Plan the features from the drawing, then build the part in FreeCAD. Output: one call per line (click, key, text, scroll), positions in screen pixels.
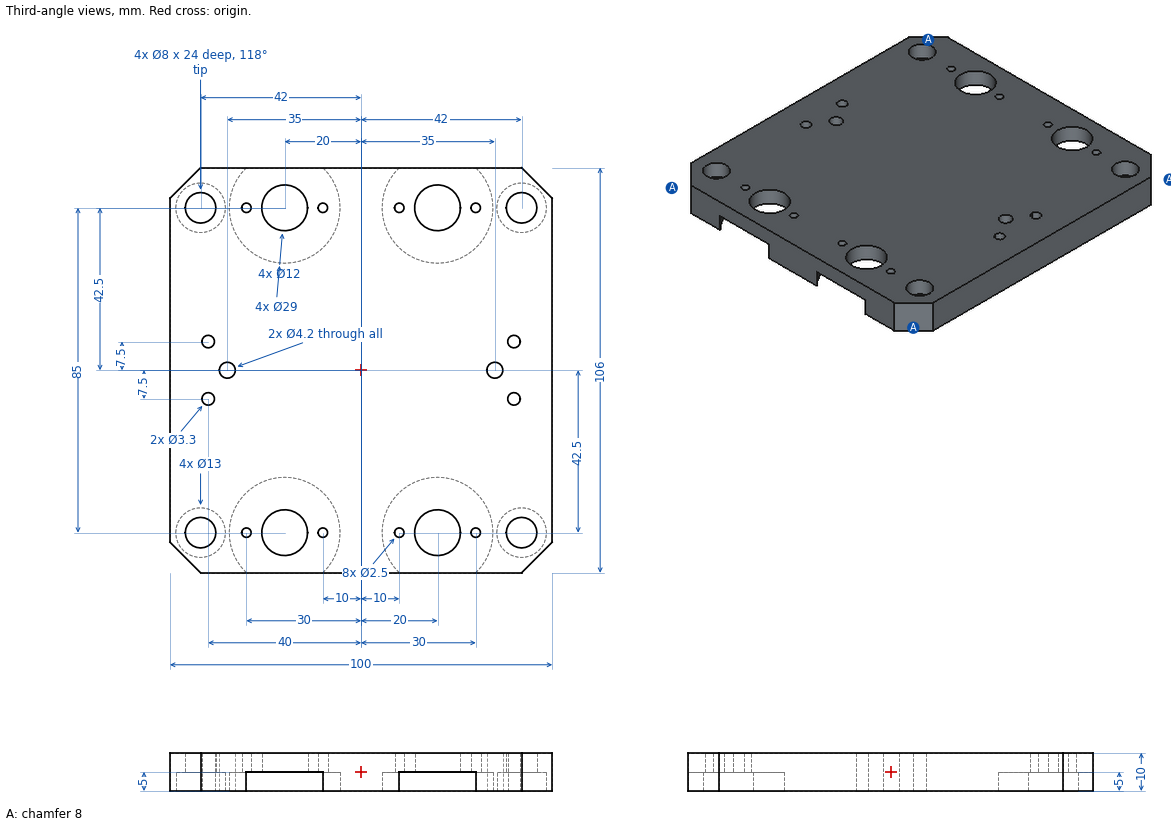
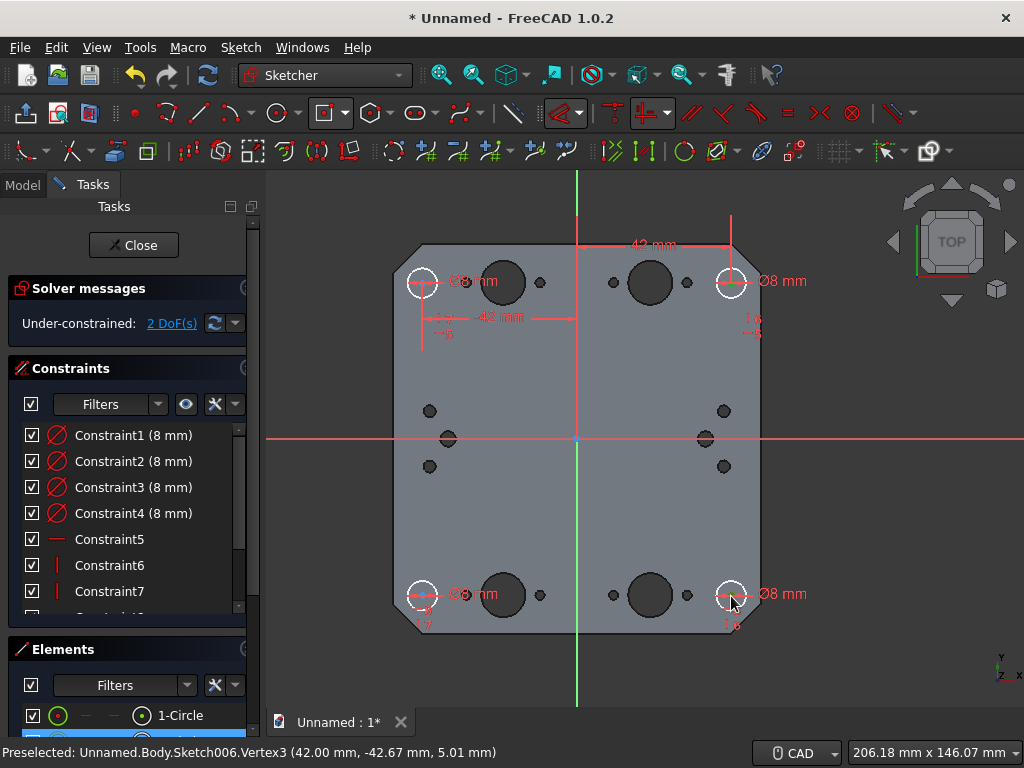
key(i)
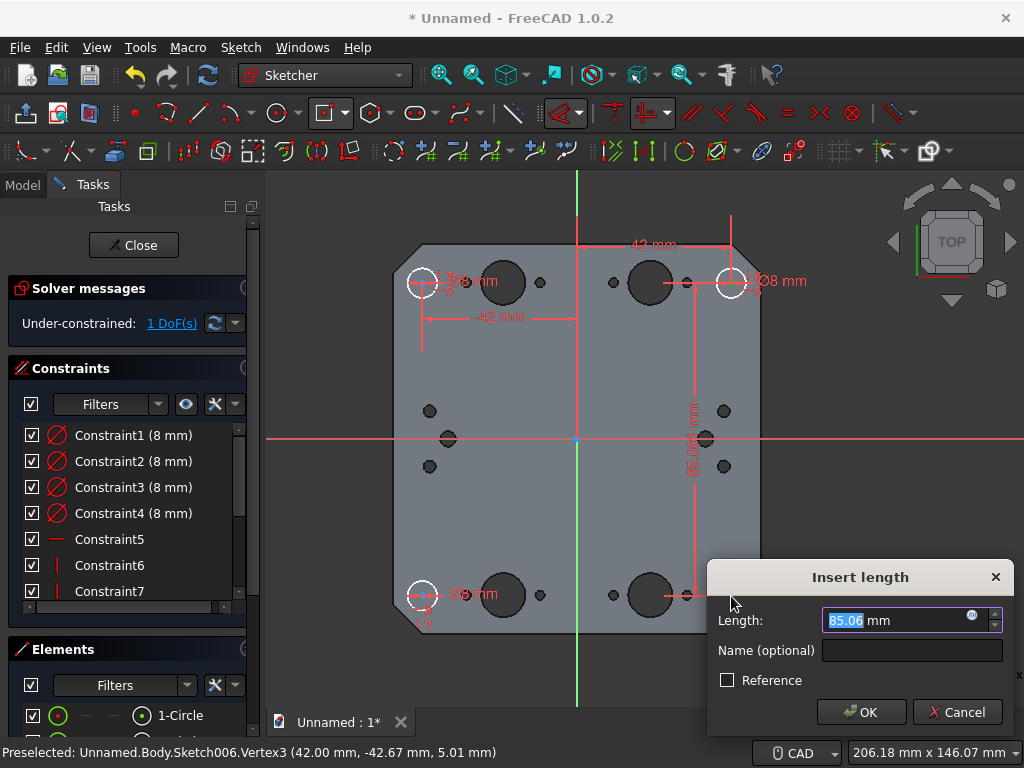
text(85)
key(Return)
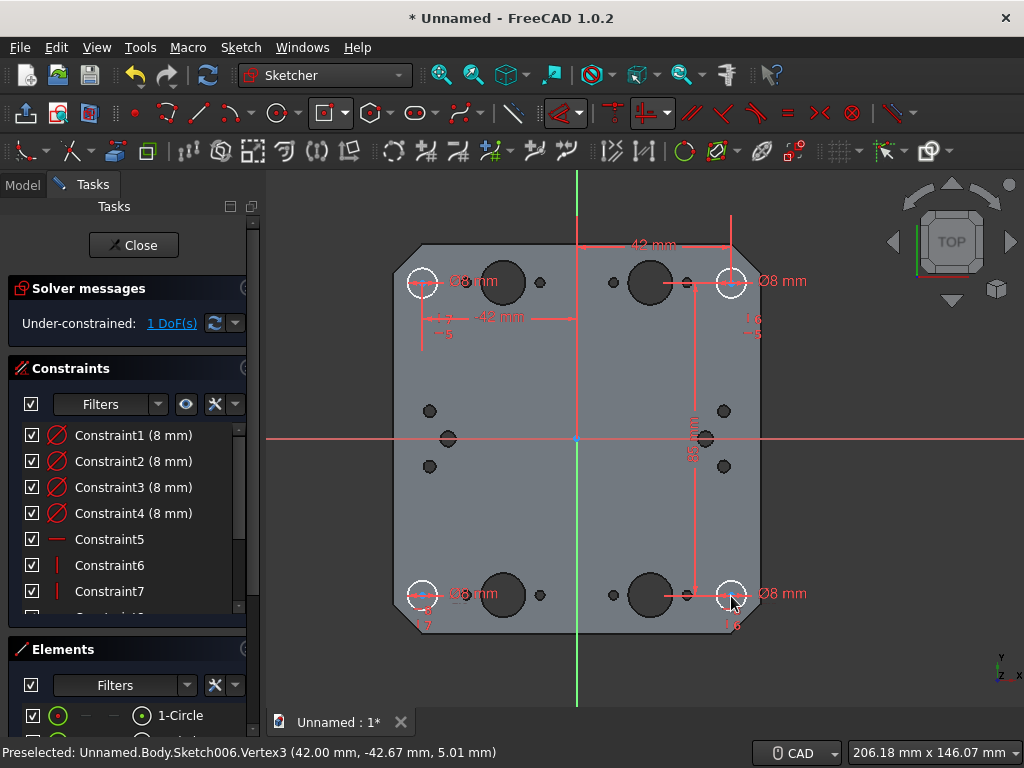
click(422, 283)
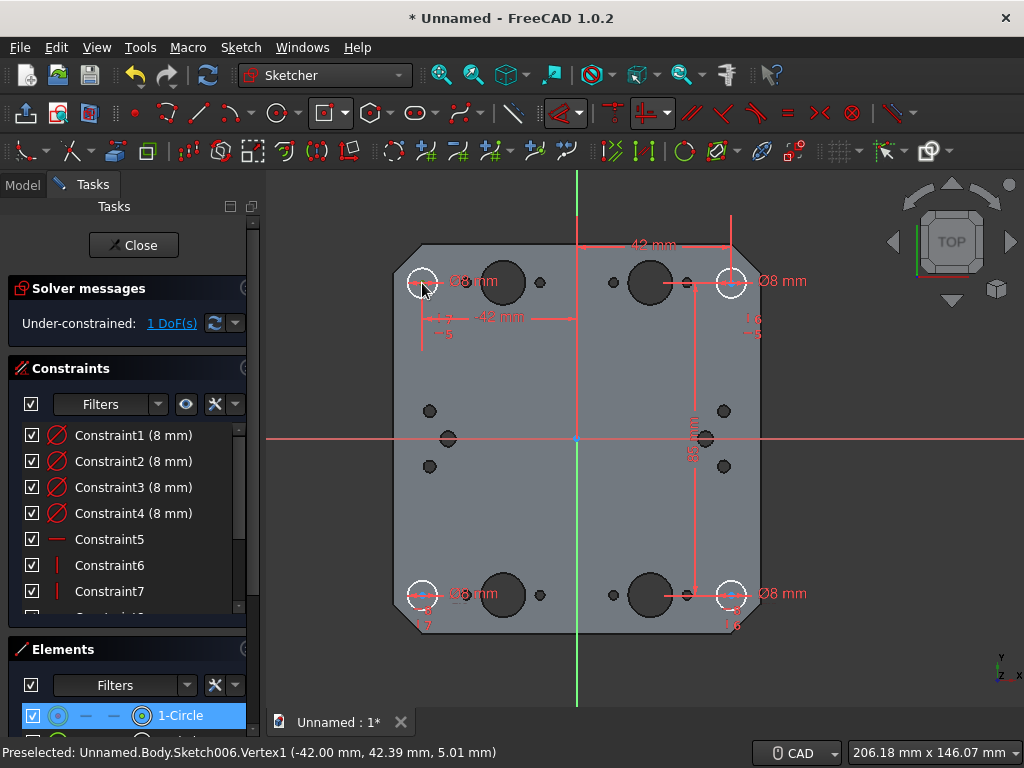
click(582, 114)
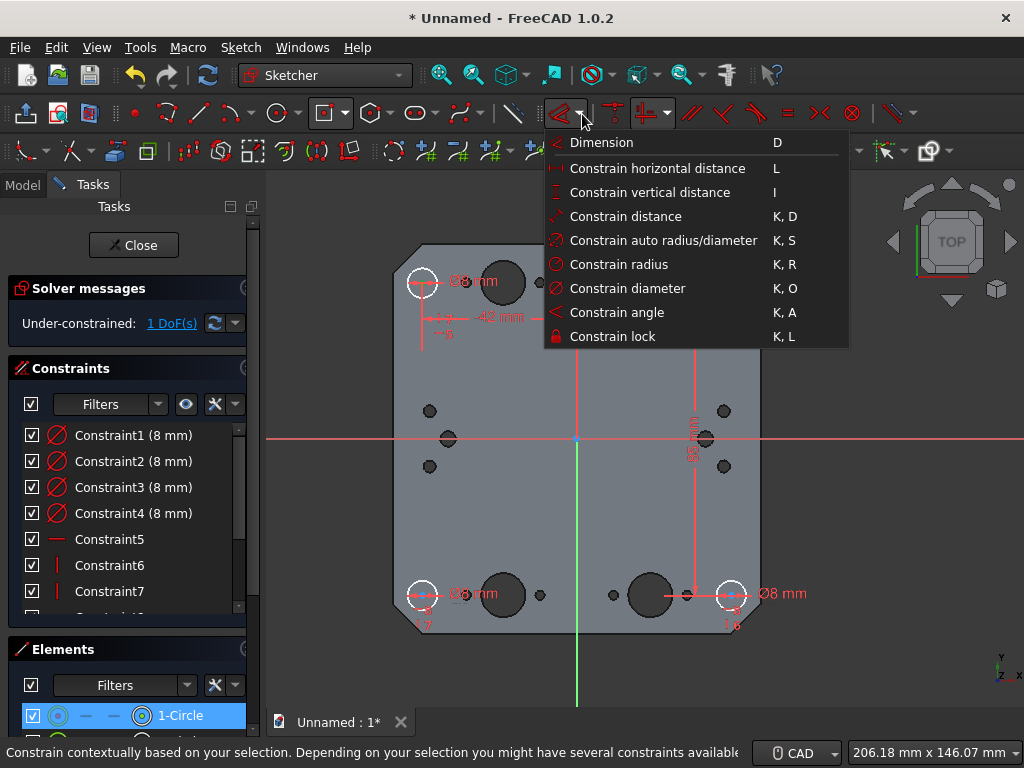
click(697, 192)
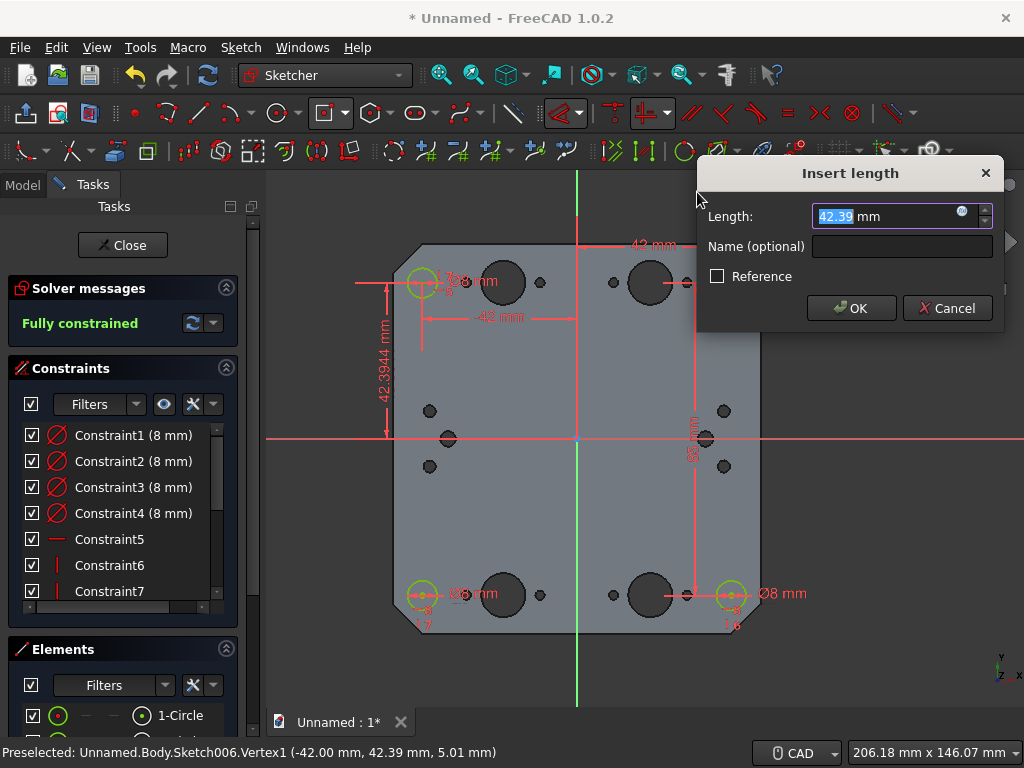
text(42.5)
key(Return)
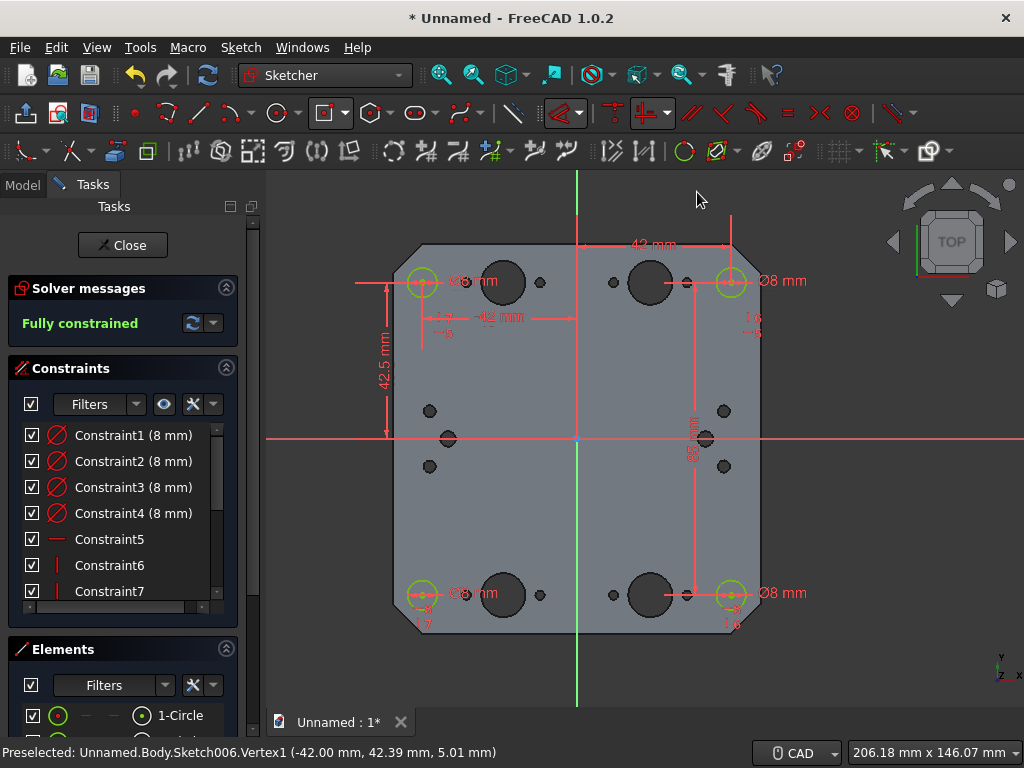
click(123, 245)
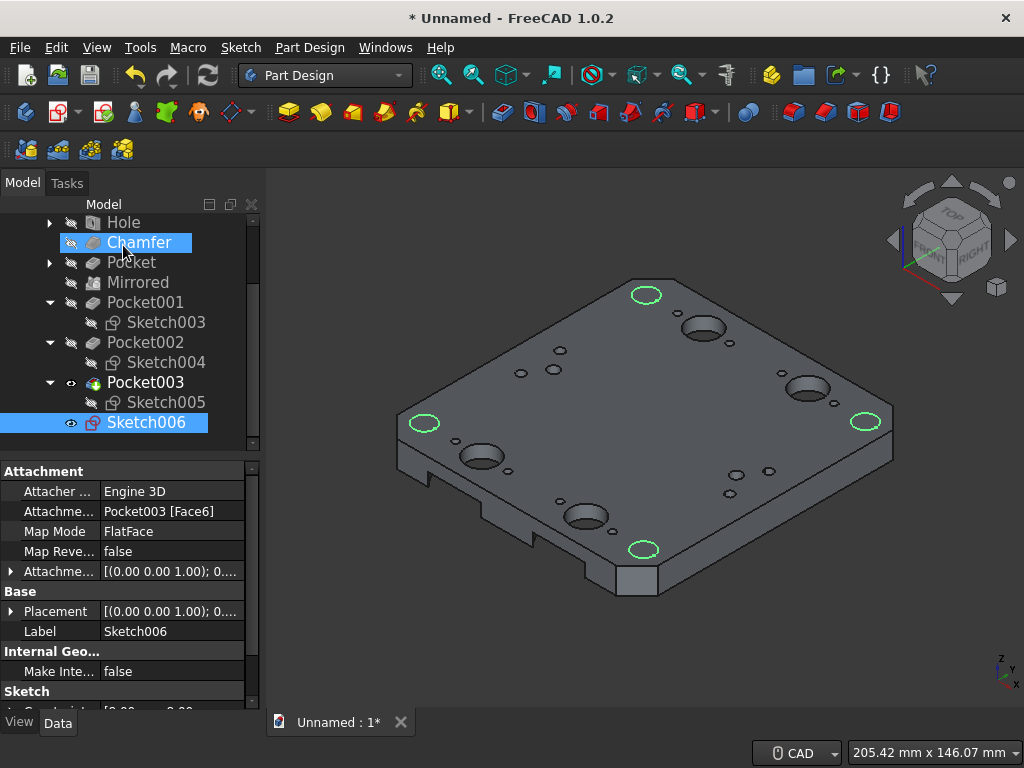
click(536, 112)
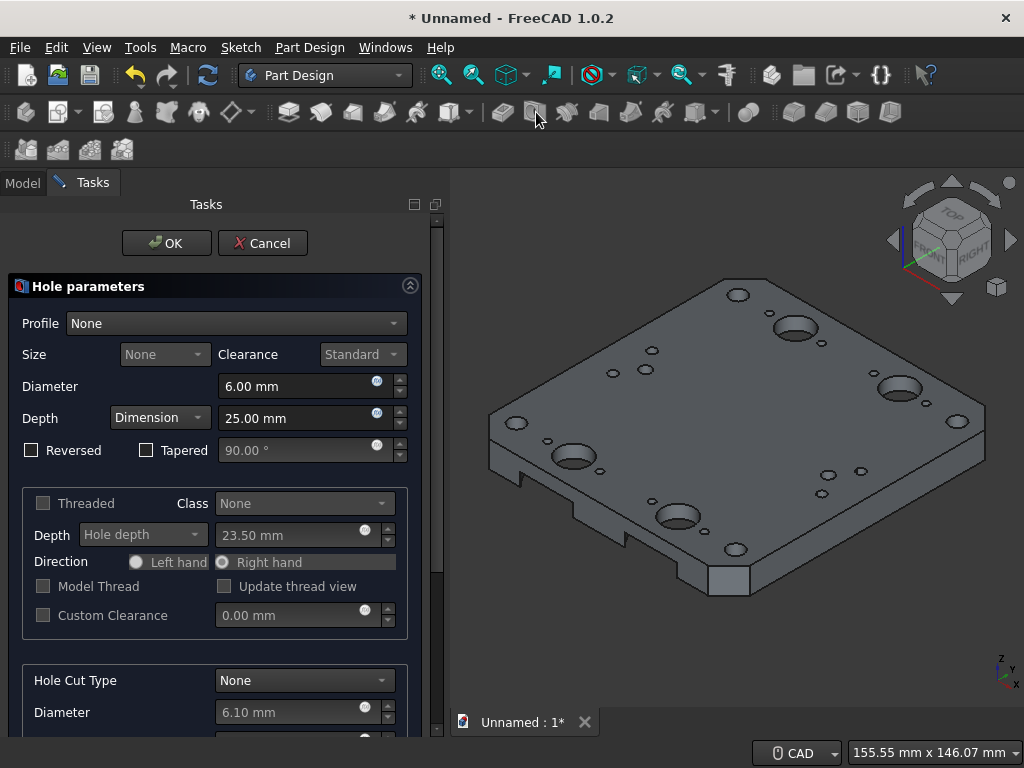
triple_click(305, 386)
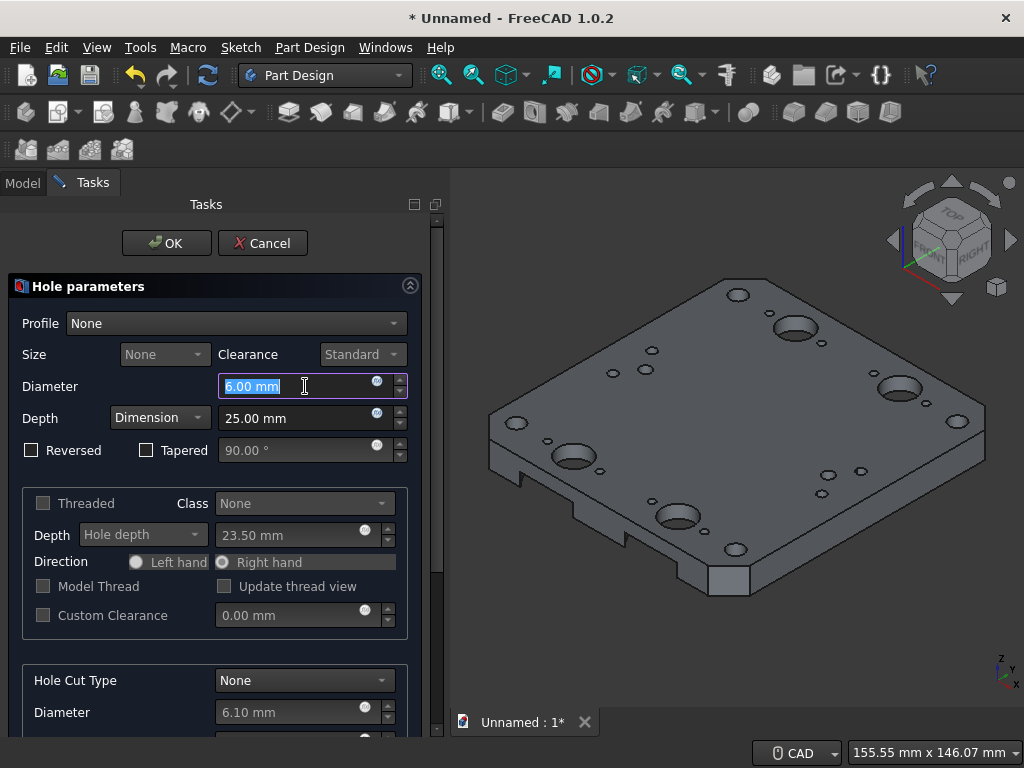
text(8)
key(Tab)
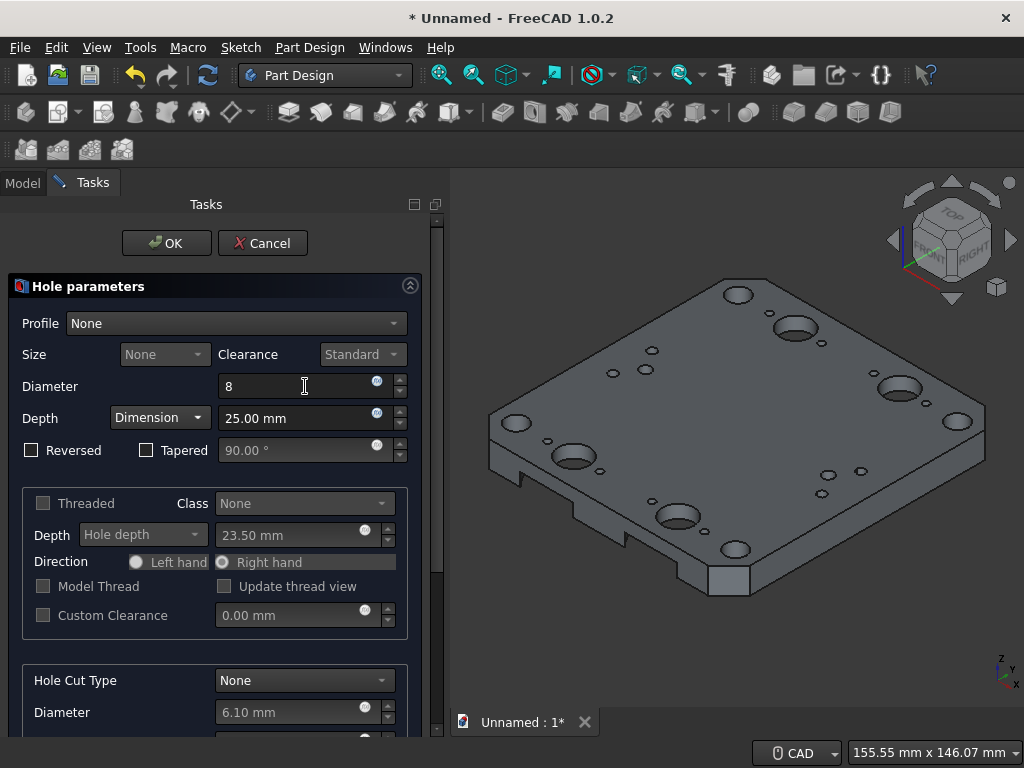
triple_click(305, 418)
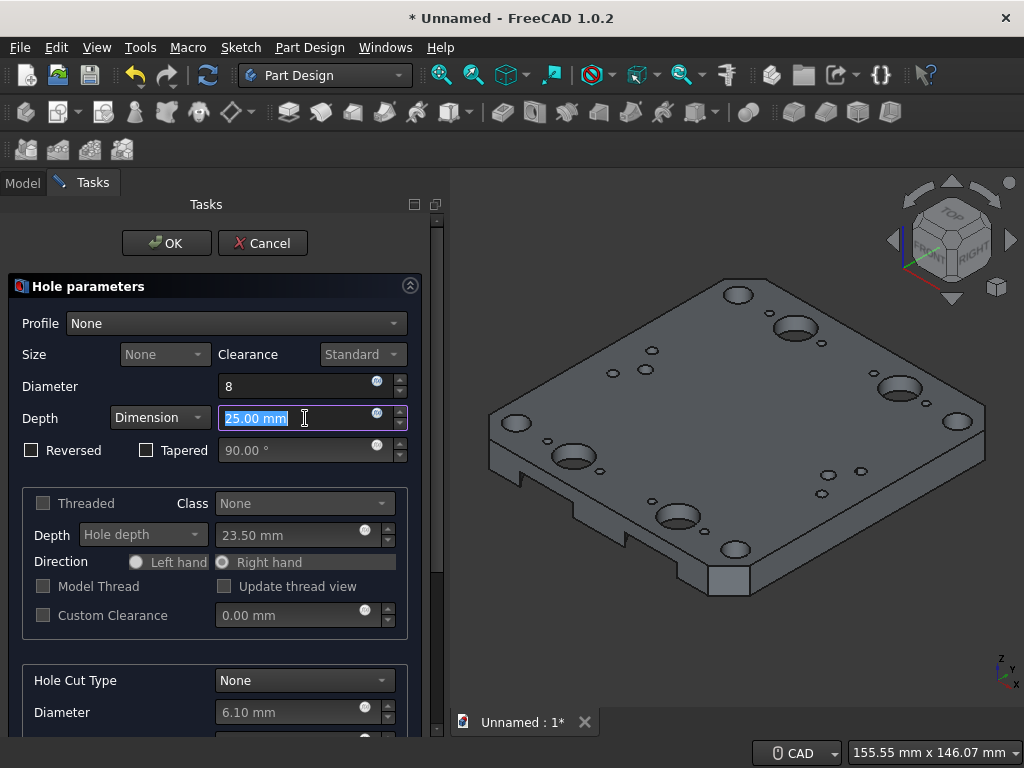
text(24)
key(Tab)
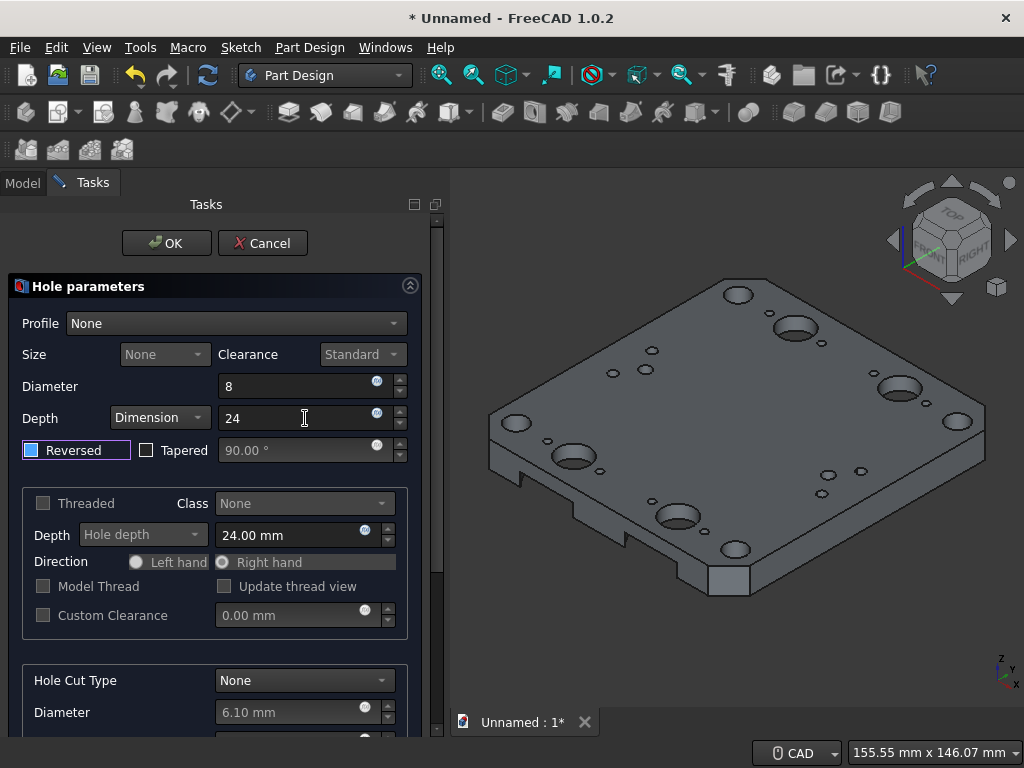
click(167, 243)